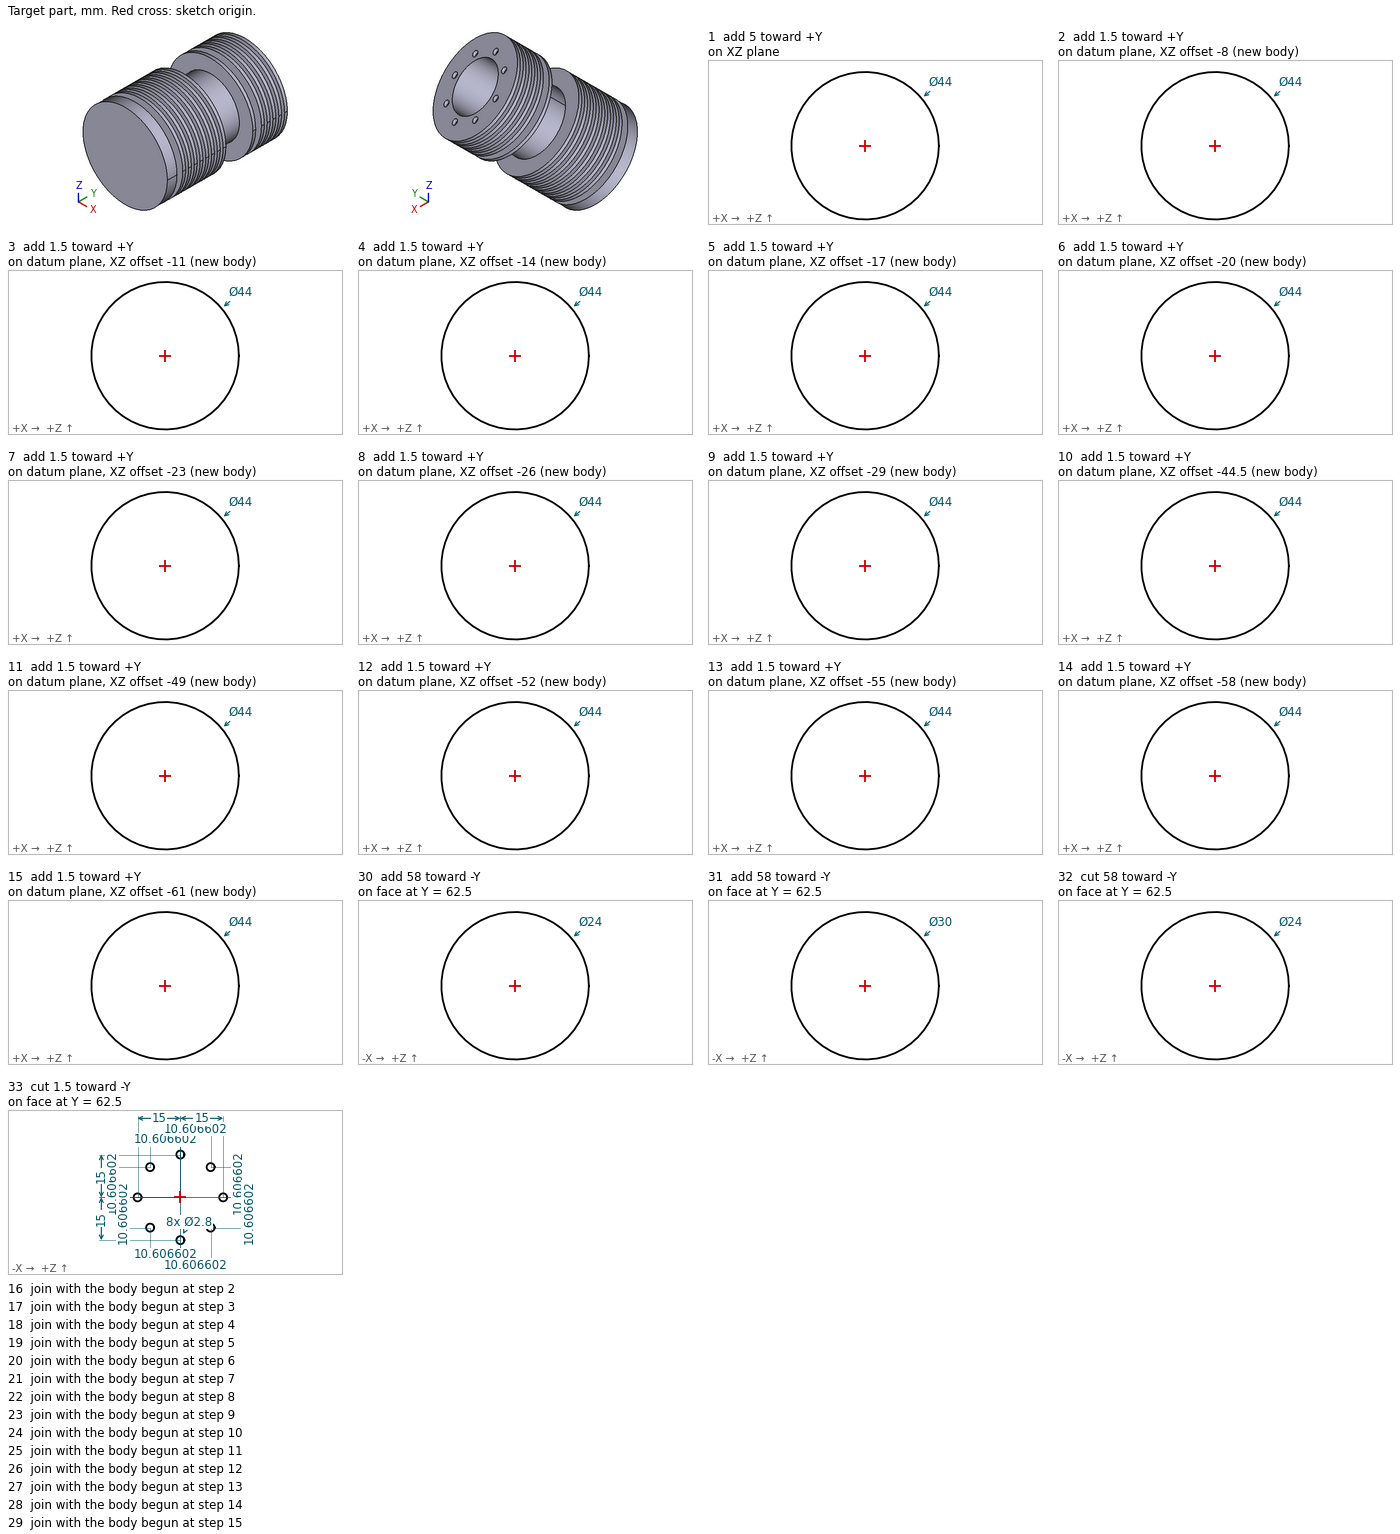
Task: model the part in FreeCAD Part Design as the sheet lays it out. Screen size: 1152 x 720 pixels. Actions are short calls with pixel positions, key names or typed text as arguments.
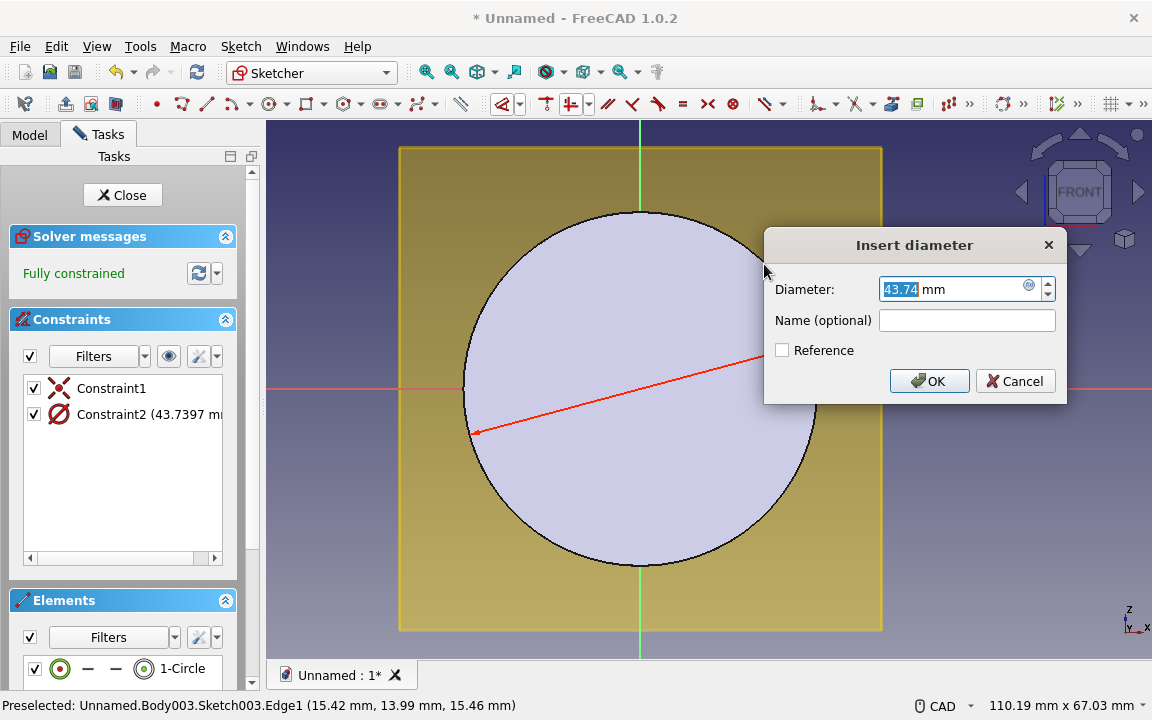
text(44)
key(Return)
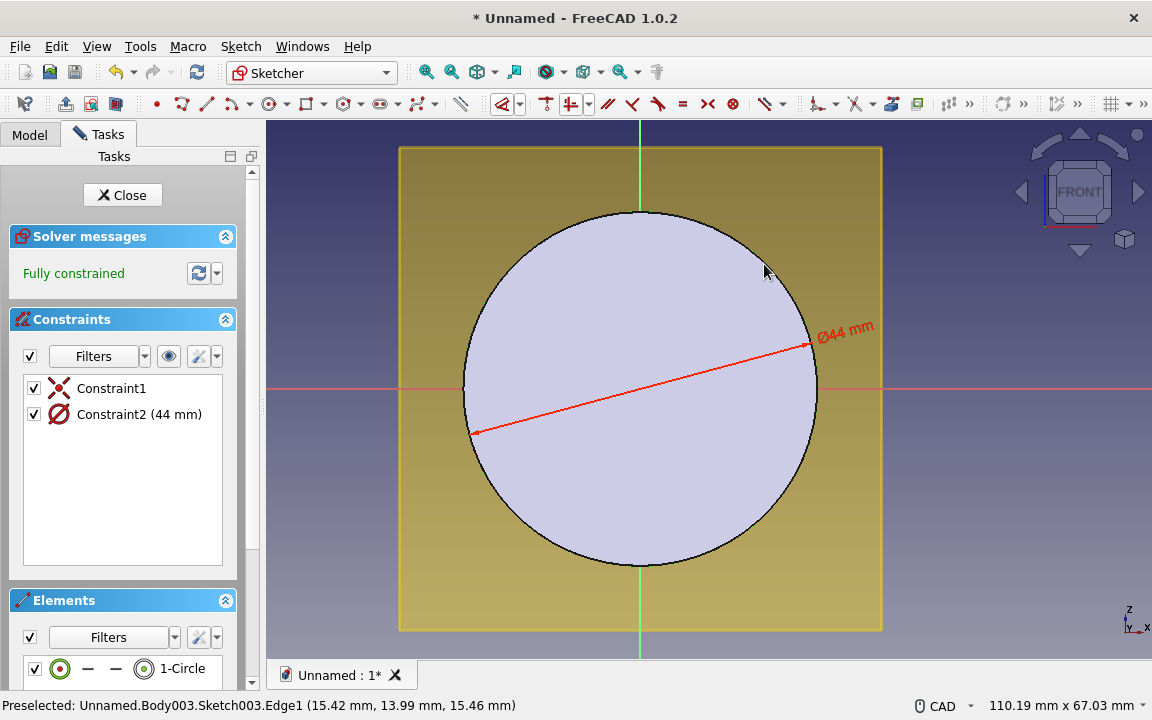
click(123, 195)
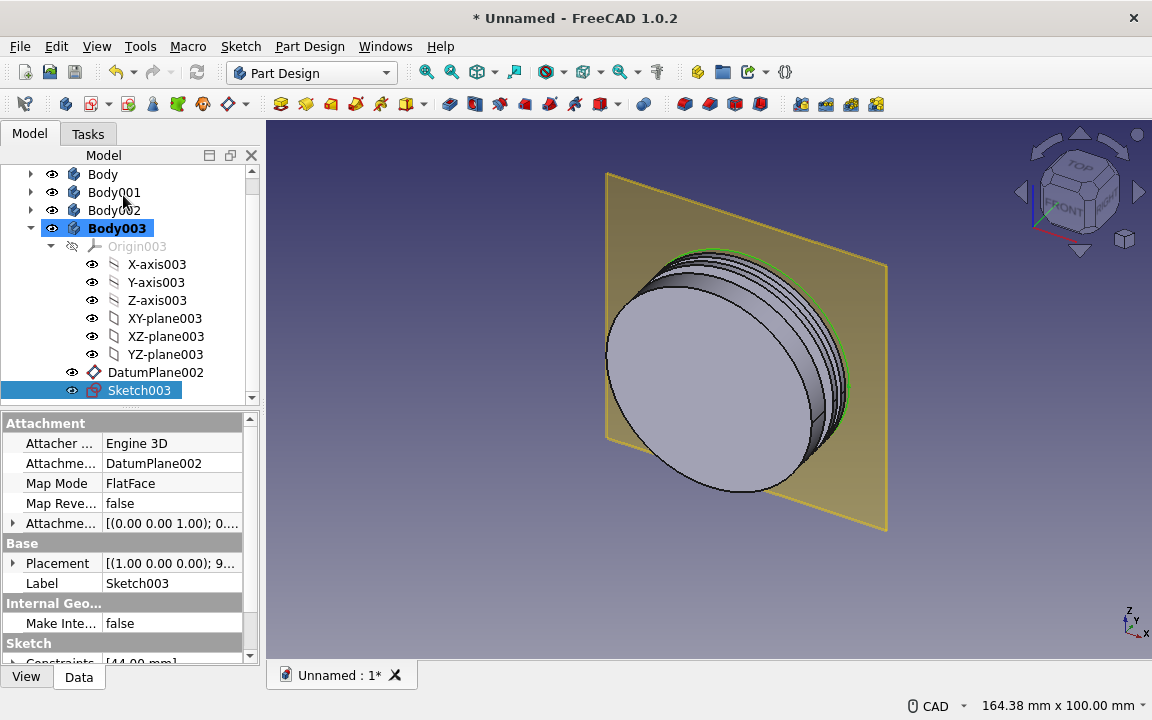
click(281, 104)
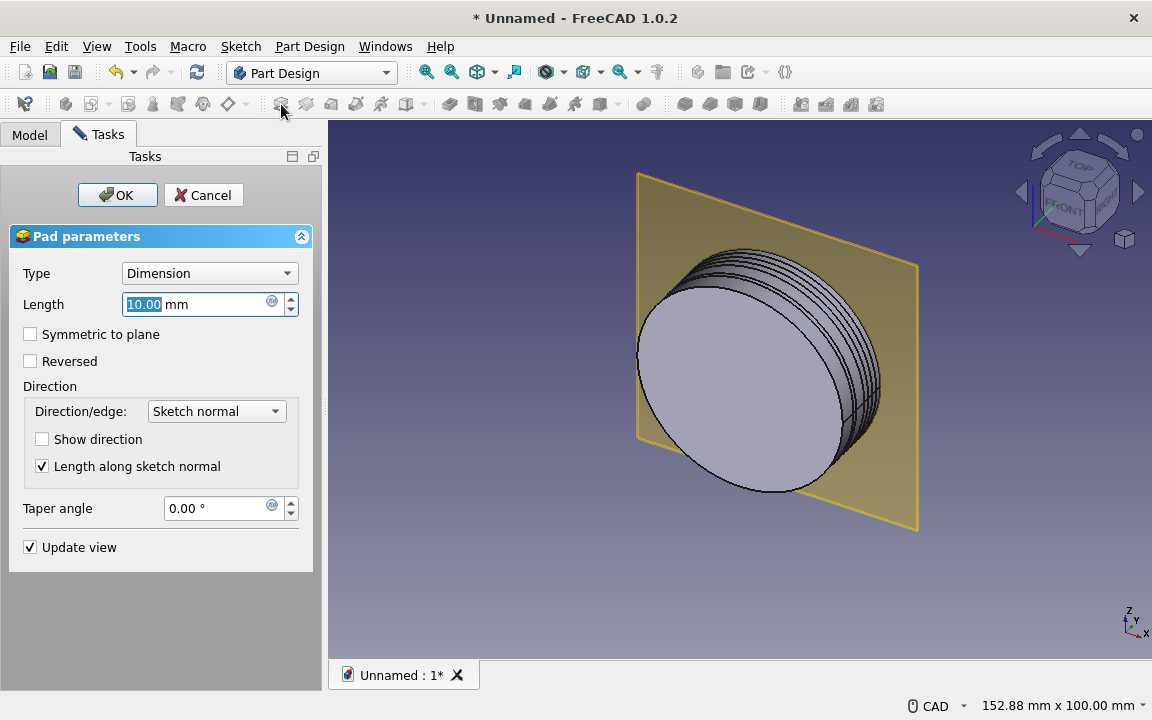
text(1.5)
key(Tab)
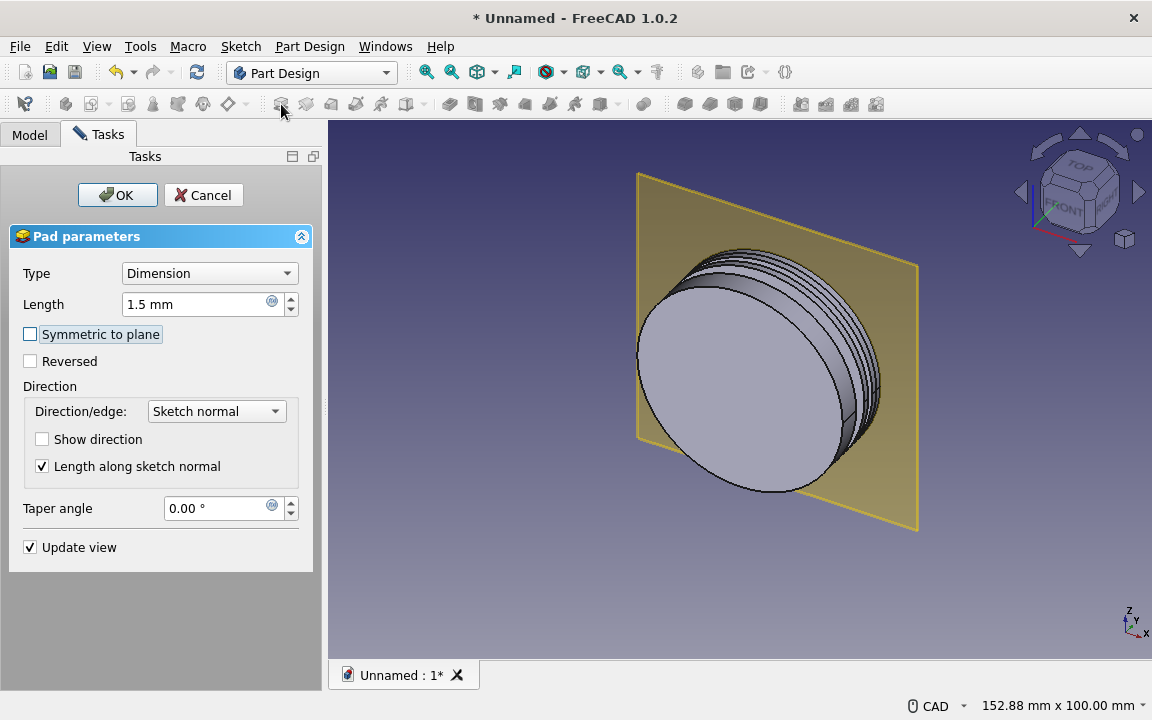
click(31, 361)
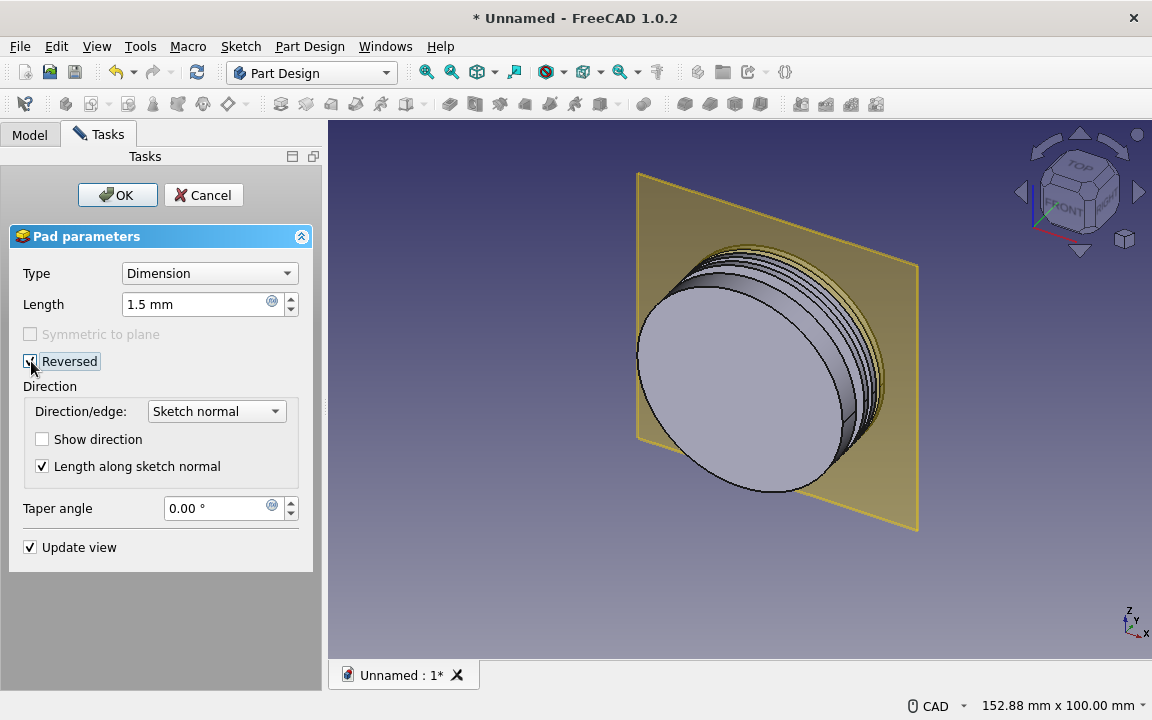
click(118, 195)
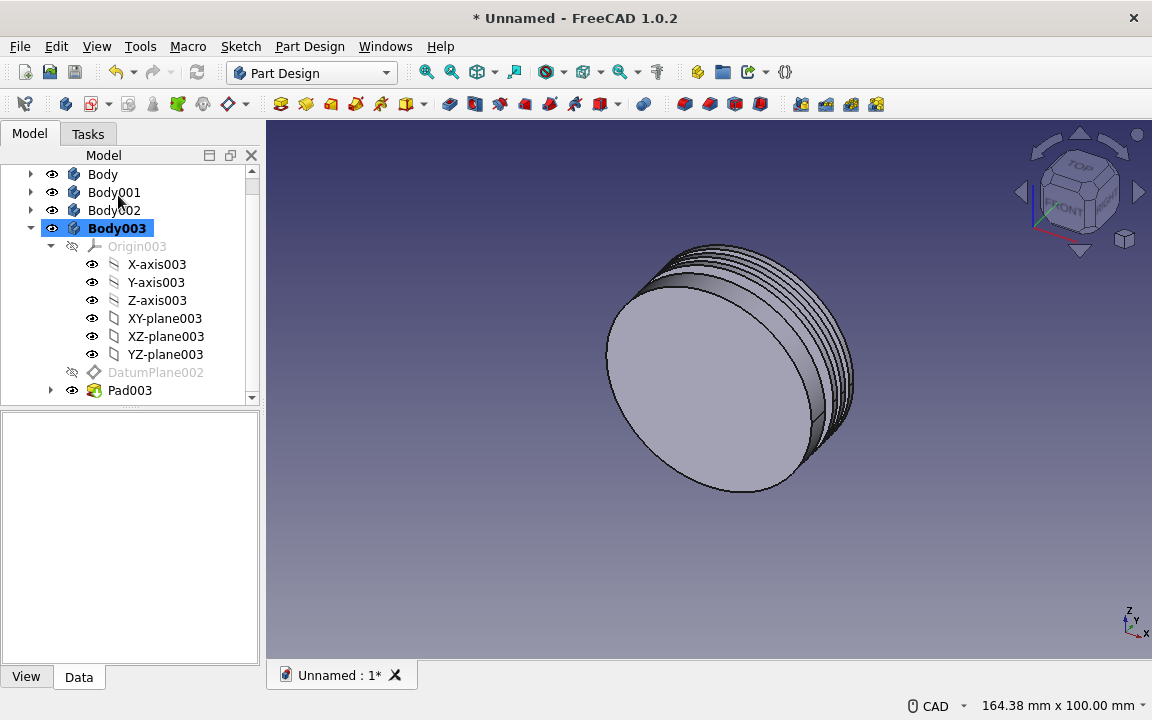
click(66, 104)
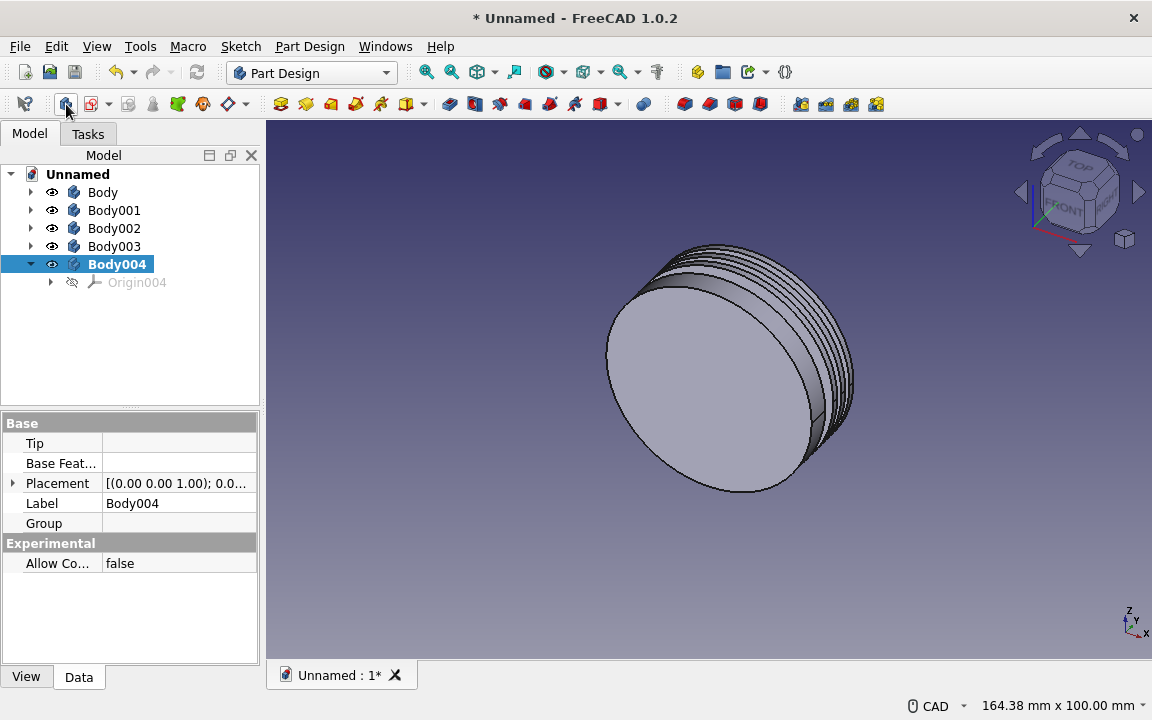
click(51, 282)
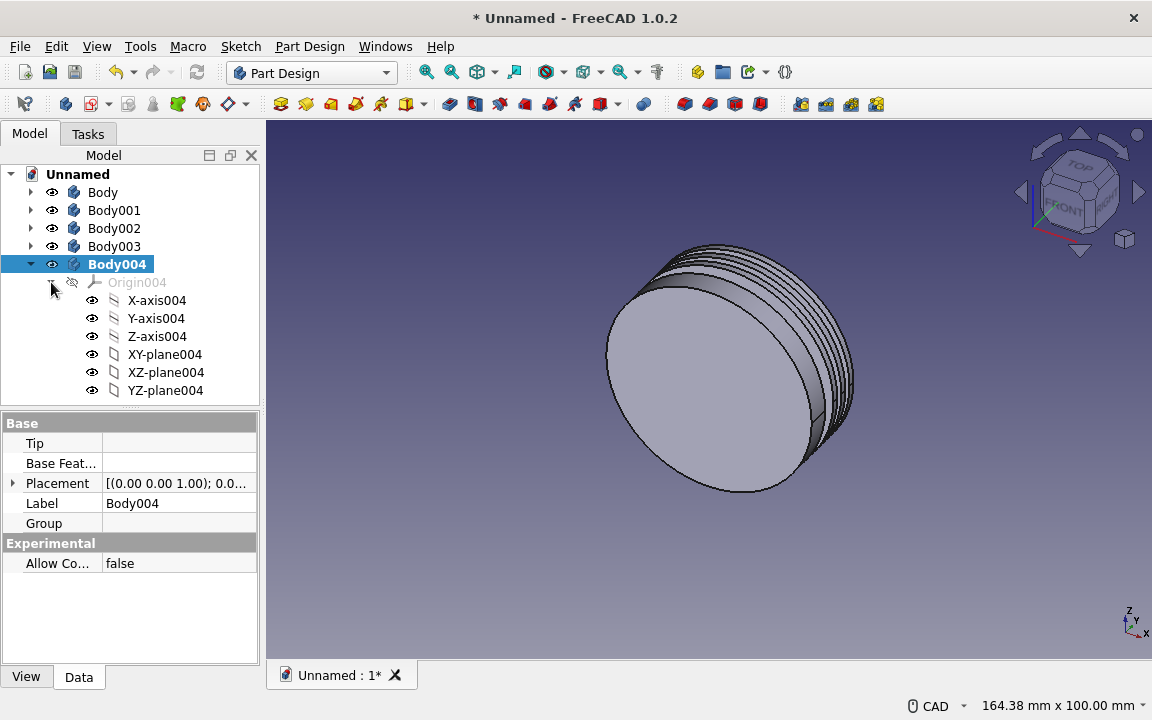
click(137, 372)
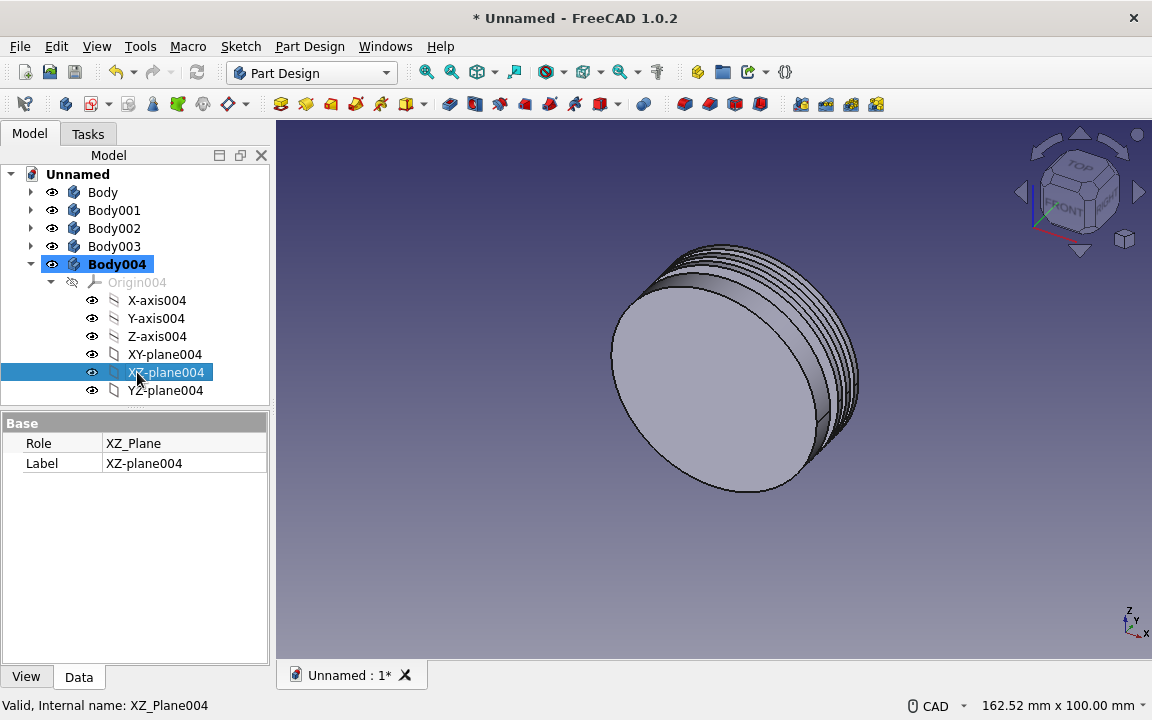
click(228, 104)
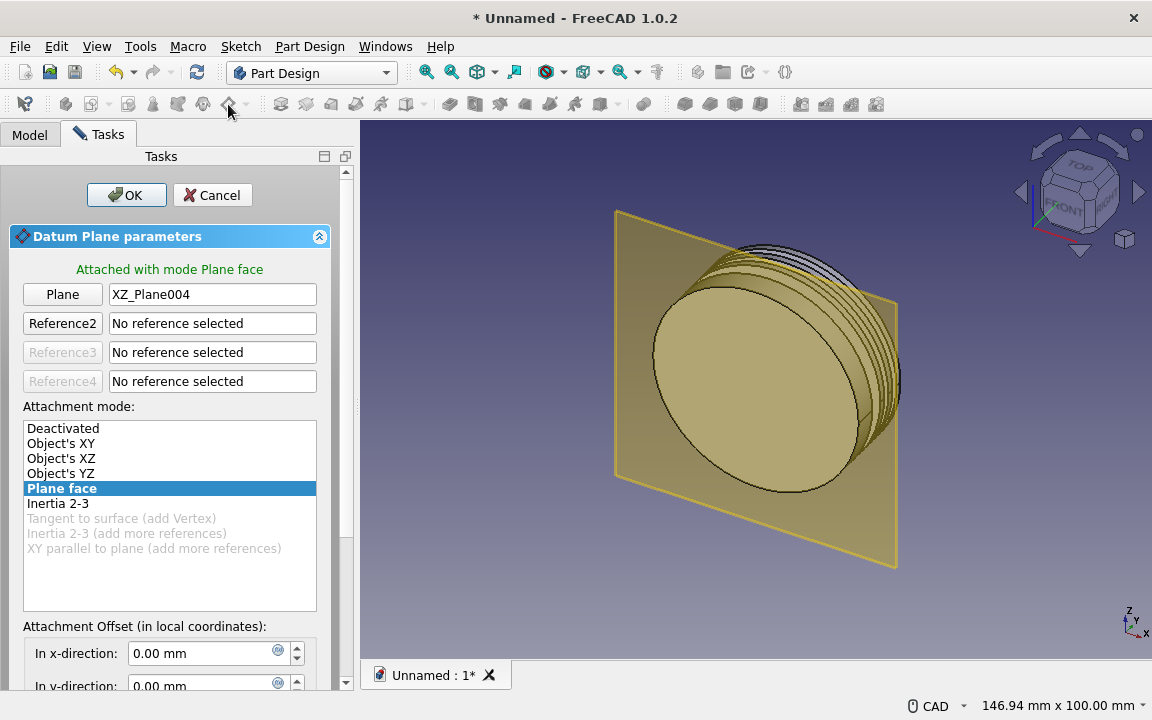
scroll(346, 428, down, 2)